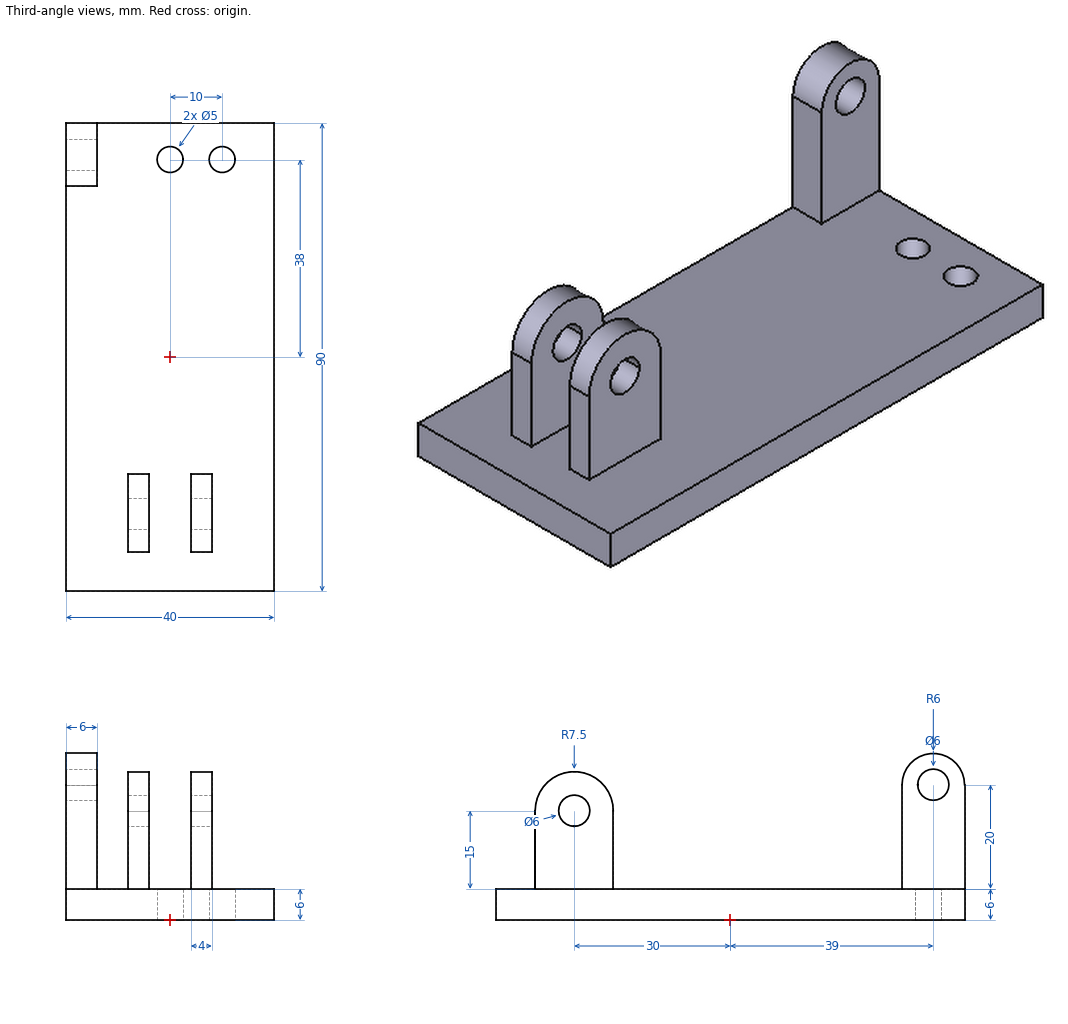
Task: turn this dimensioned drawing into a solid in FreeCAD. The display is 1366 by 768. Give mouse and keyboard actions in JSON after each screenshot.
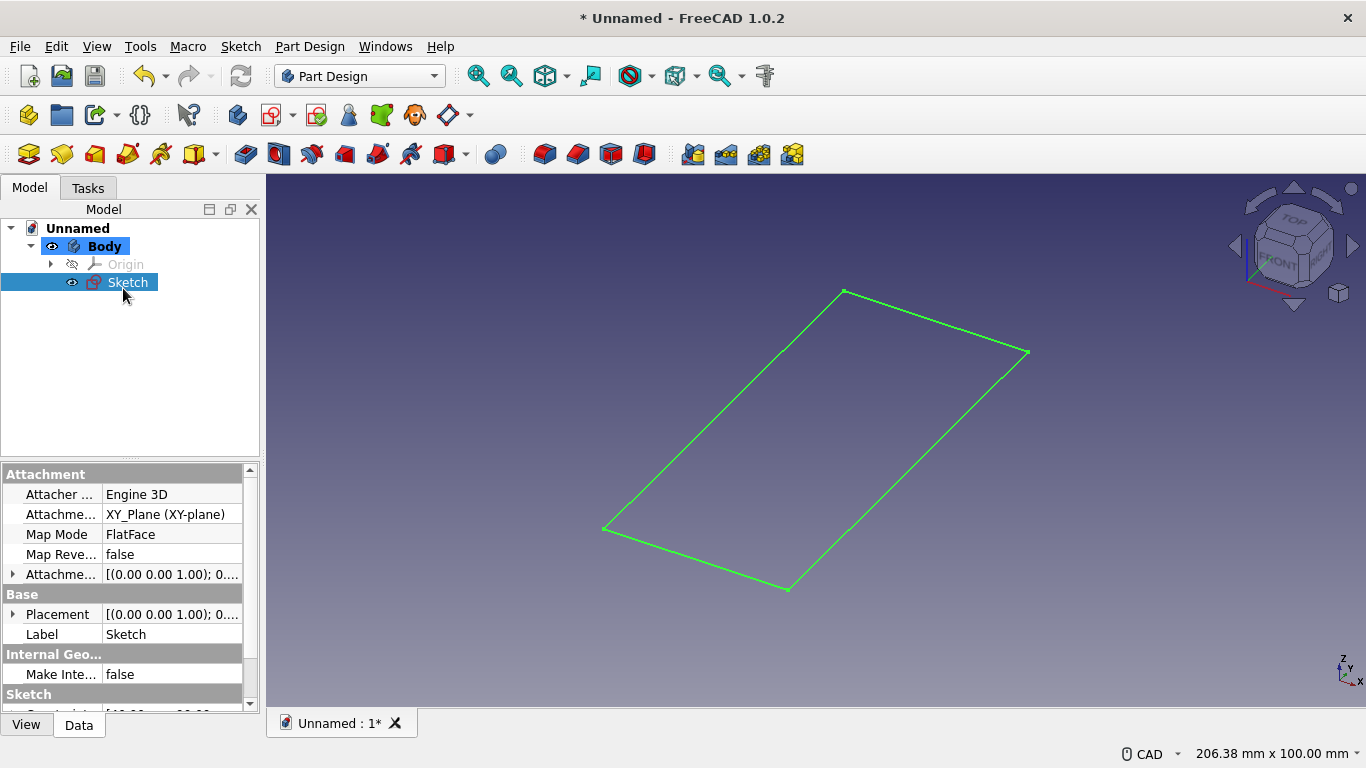
{"action": "left_click", "coordinate": [29, 154]}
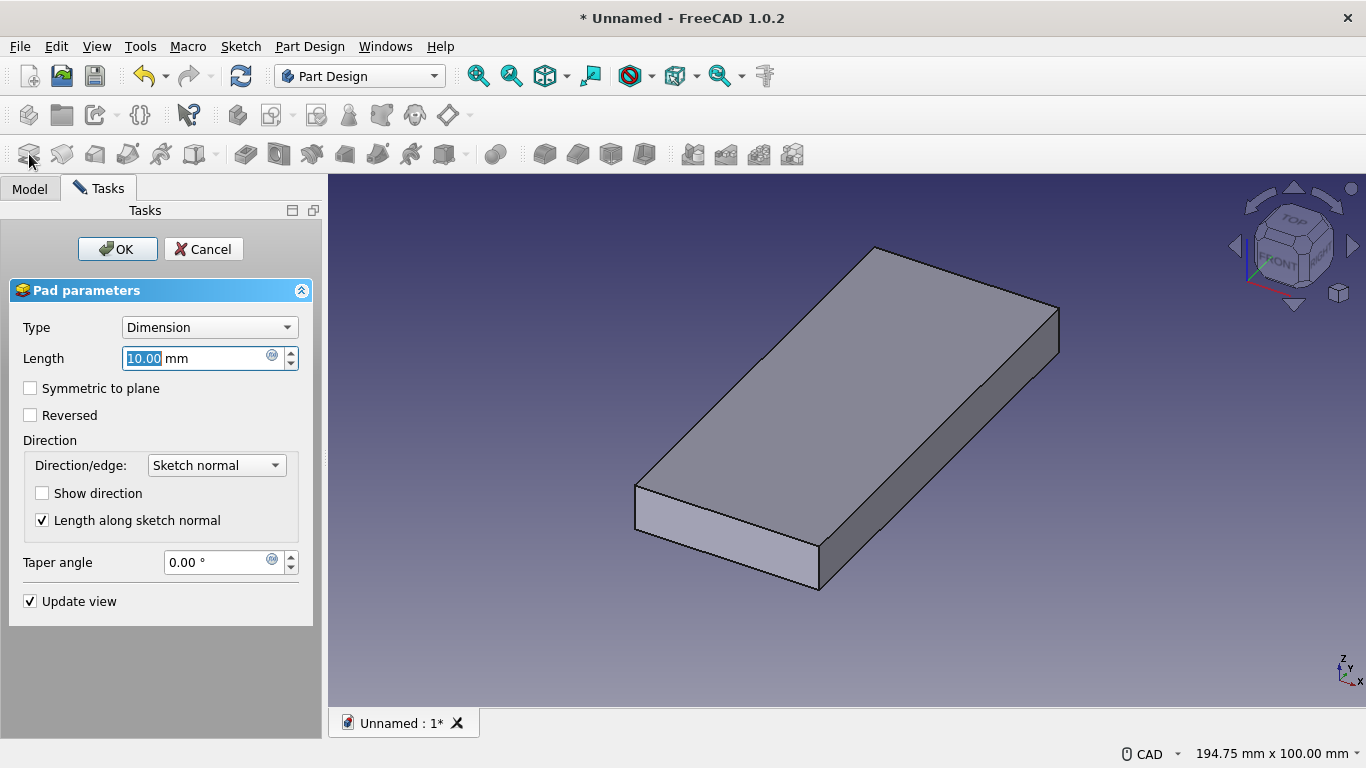
{"action": "type", "text": "6"}
{"action": "key", "text": "Tab"}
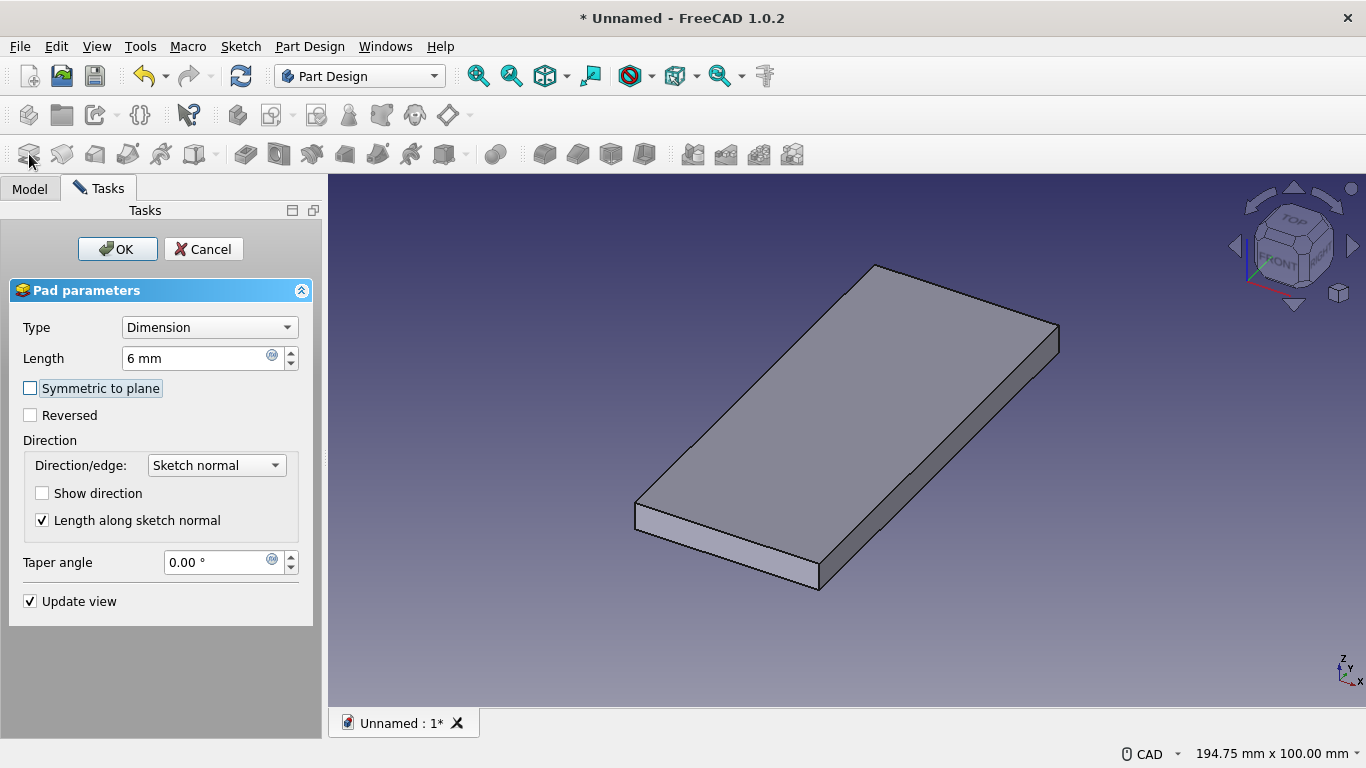
{"action": "left_click", "coordinate": [118, 249]}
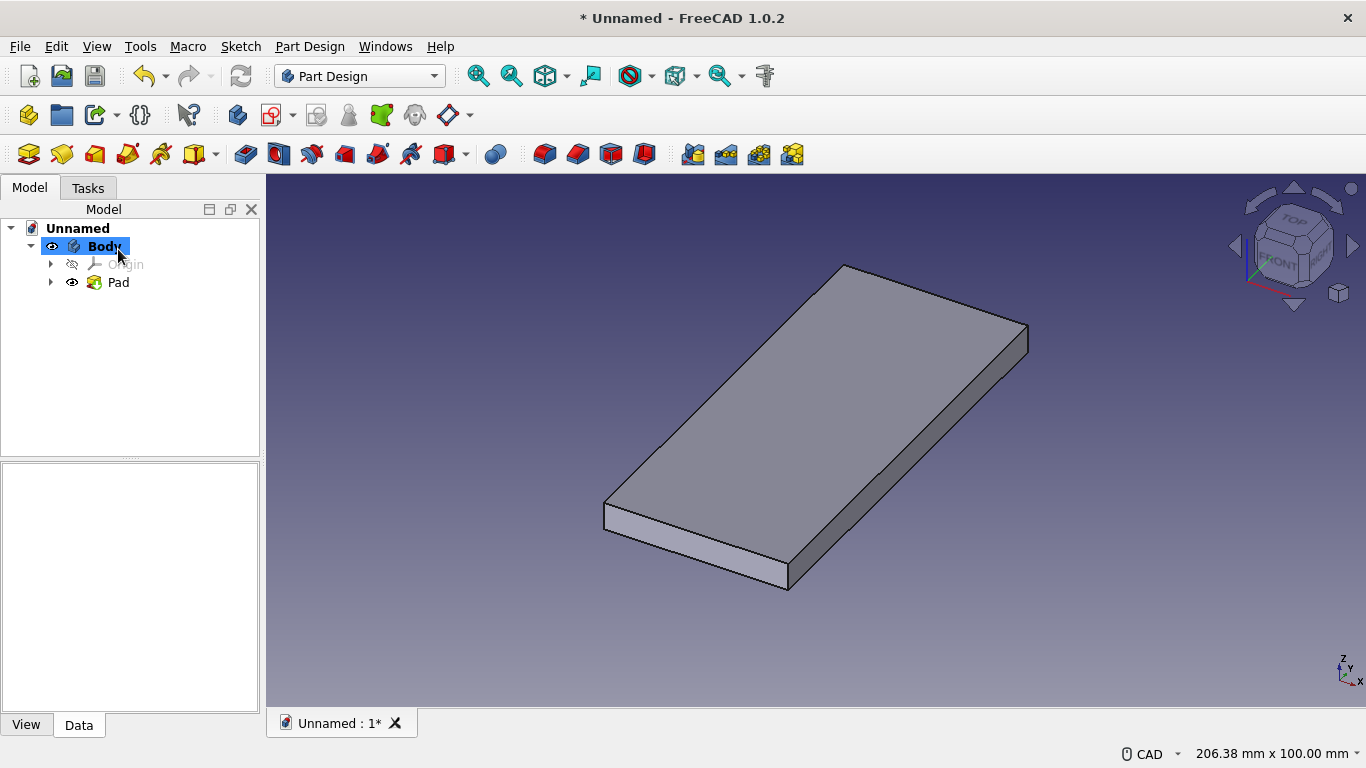
{"action": "left_click", "coordinate": [850, 379]}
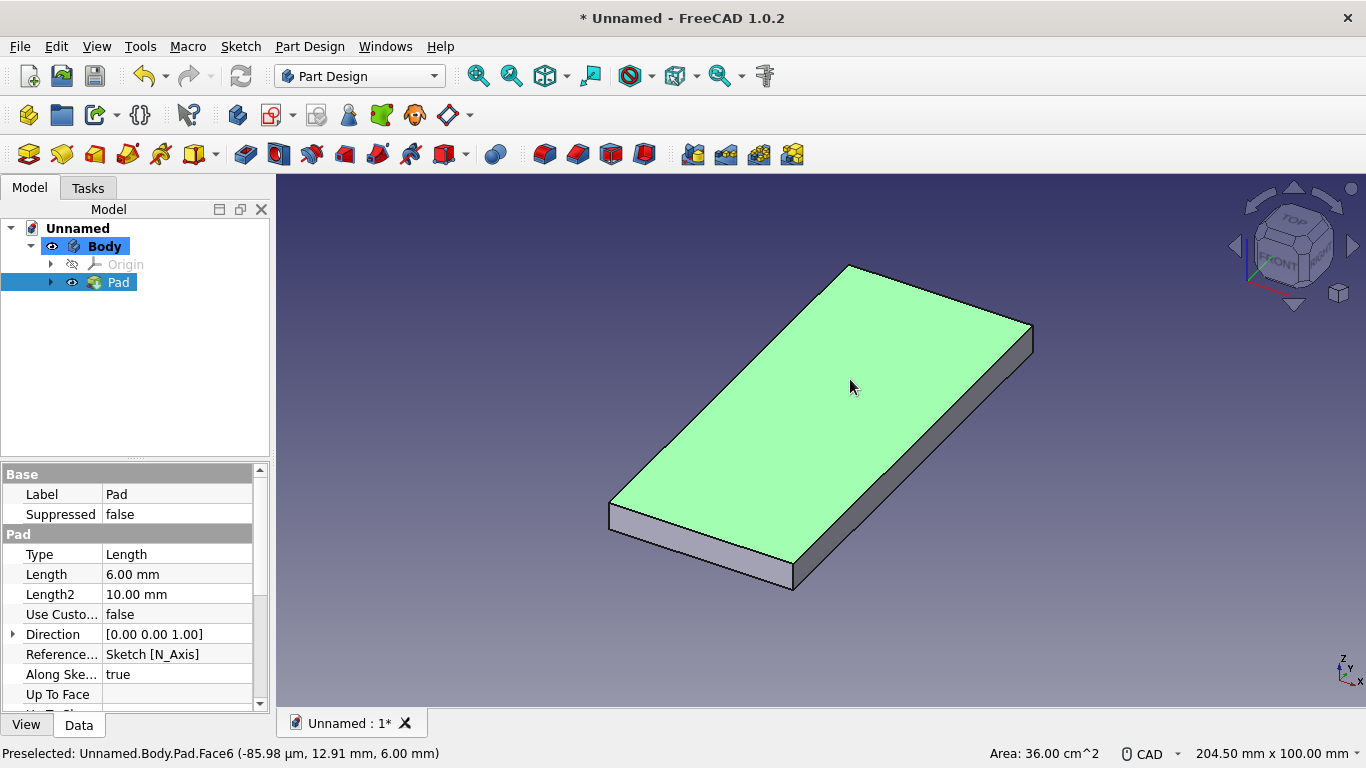
{"action": "left_click", "coordinate": [270, 116]}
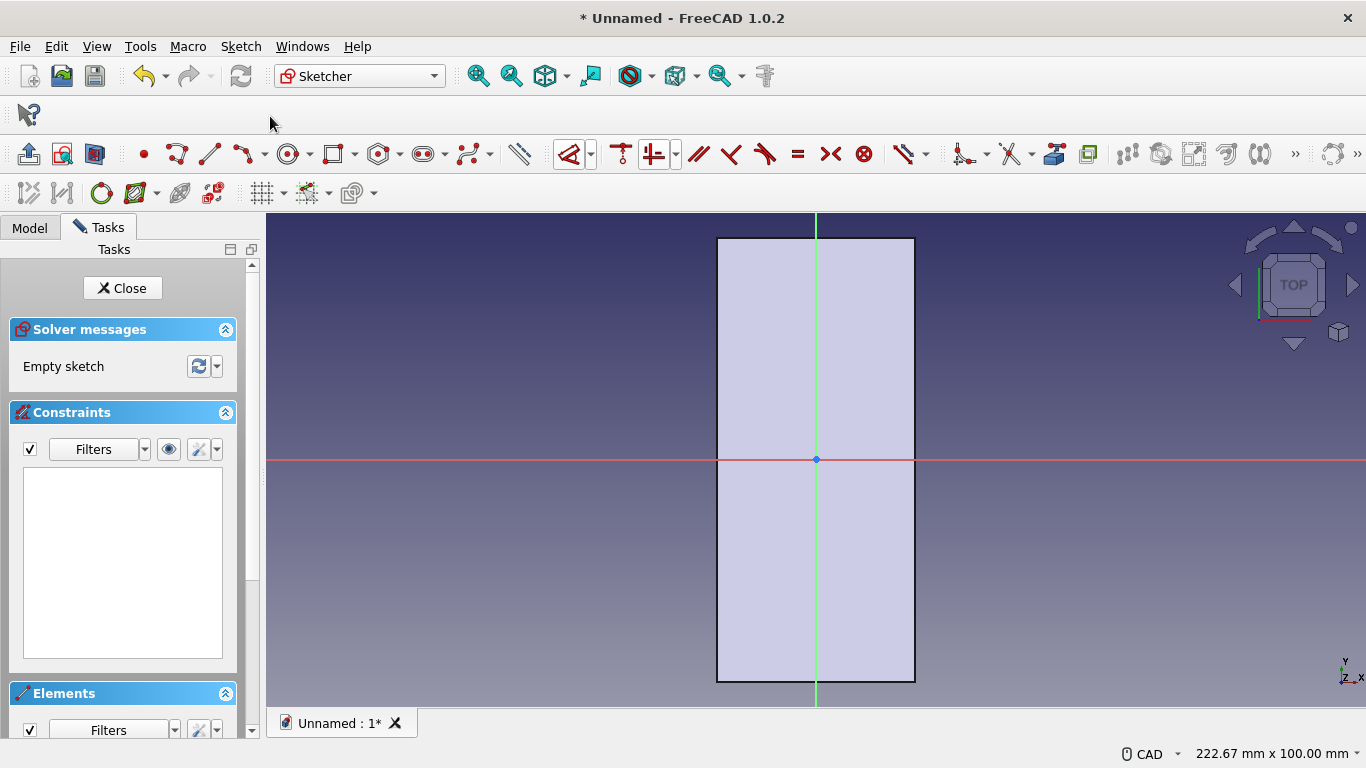
{"action": "scroll", "coordinate": [852, 249], "scroll_direction": "up", "scroll_amount": 11}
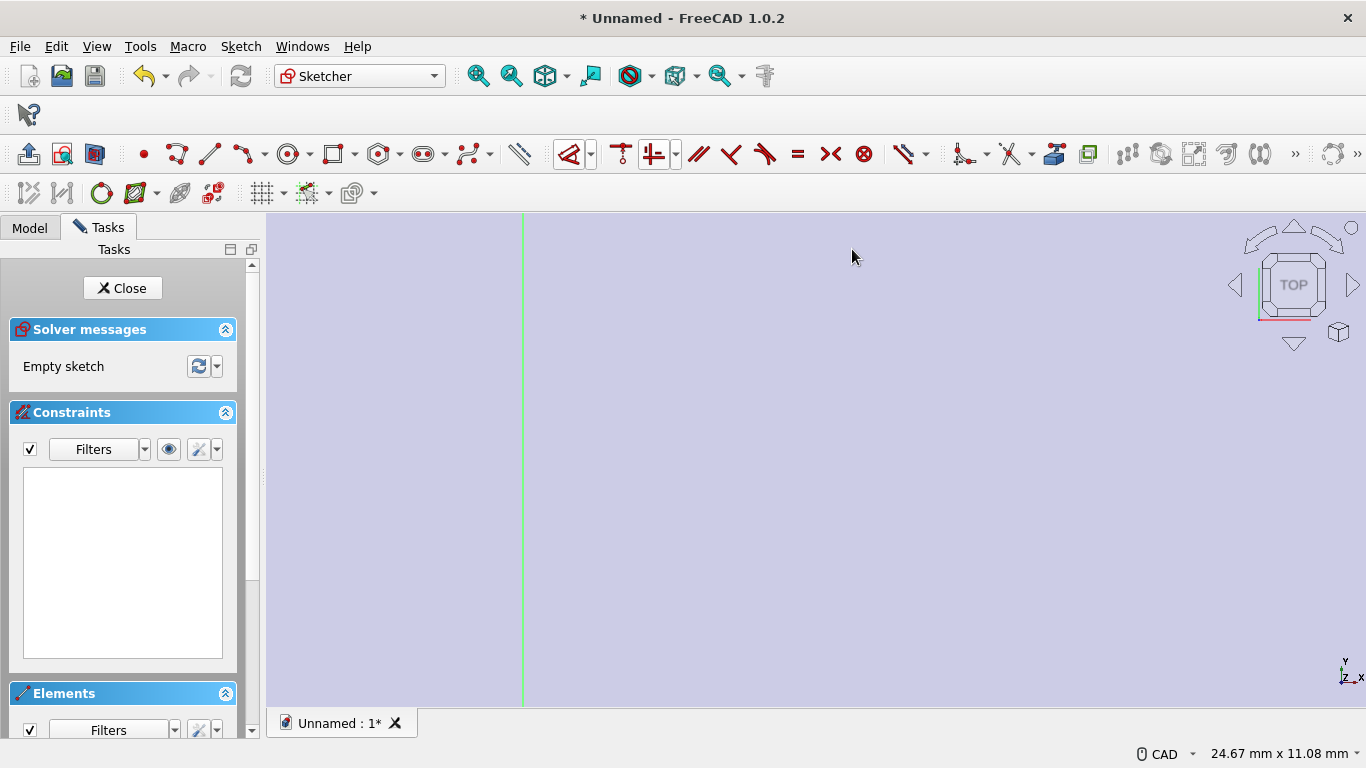
{"action": "left_click", "coordinate": [288, 154]}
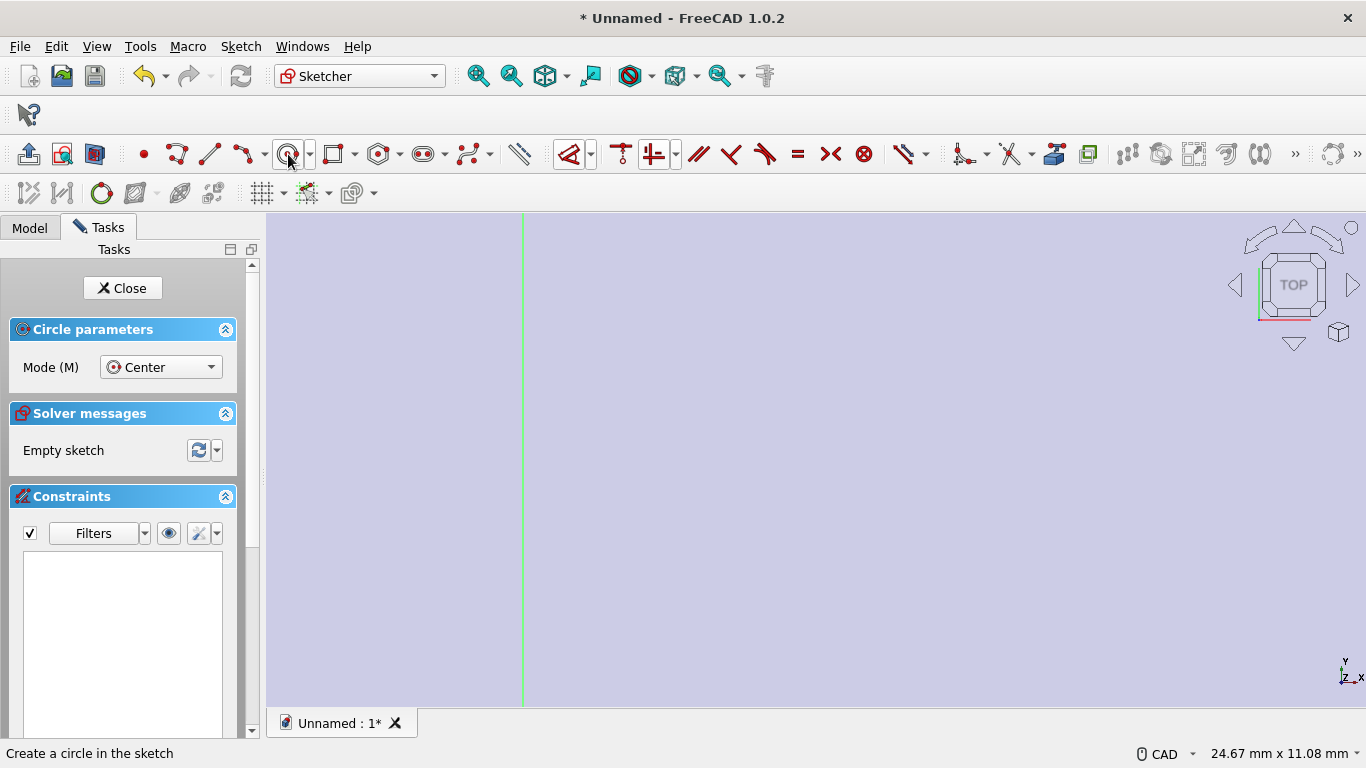
{"action": "left_click", "coordinate": [523, 459]}
{"action": "mouse_move", "coordinate": [602, 380]}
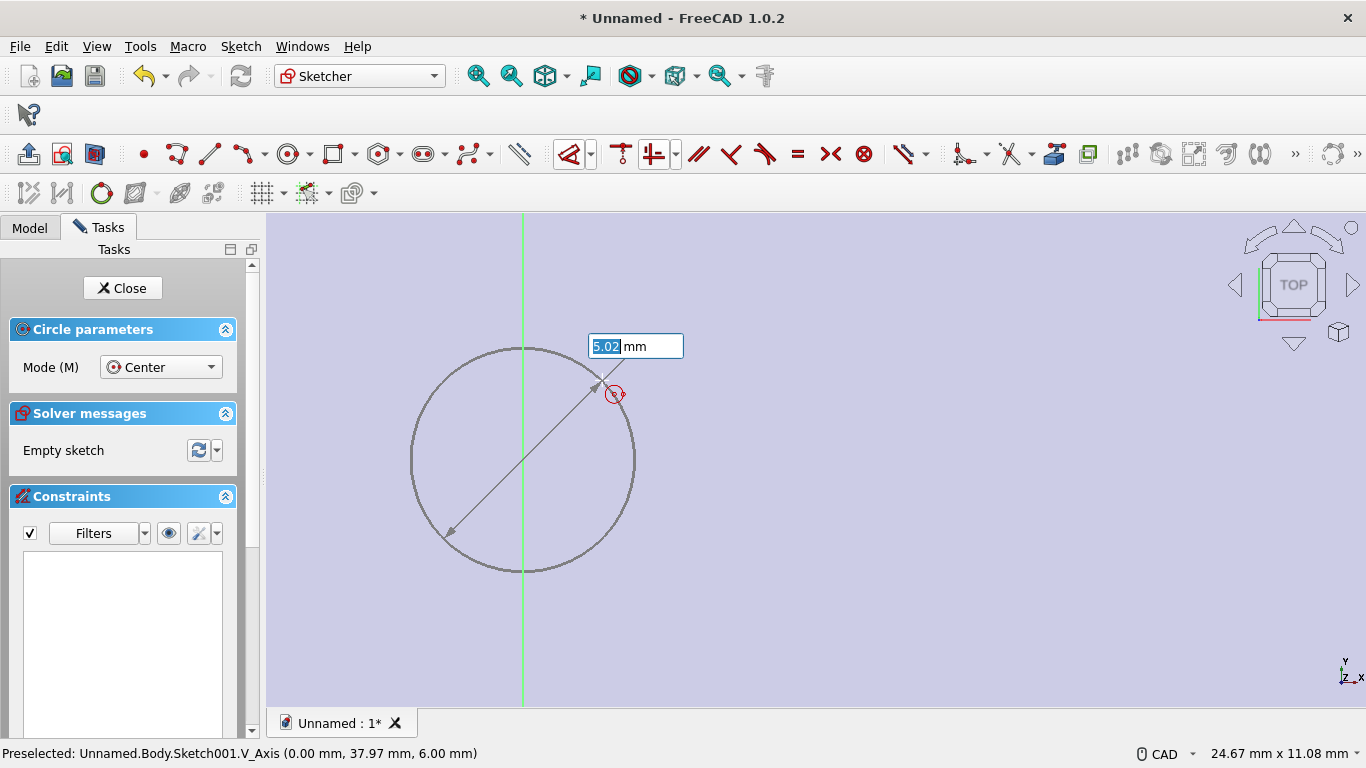
{"action": "type", "text": "5"}
{"action": "key", "text": "Return"}